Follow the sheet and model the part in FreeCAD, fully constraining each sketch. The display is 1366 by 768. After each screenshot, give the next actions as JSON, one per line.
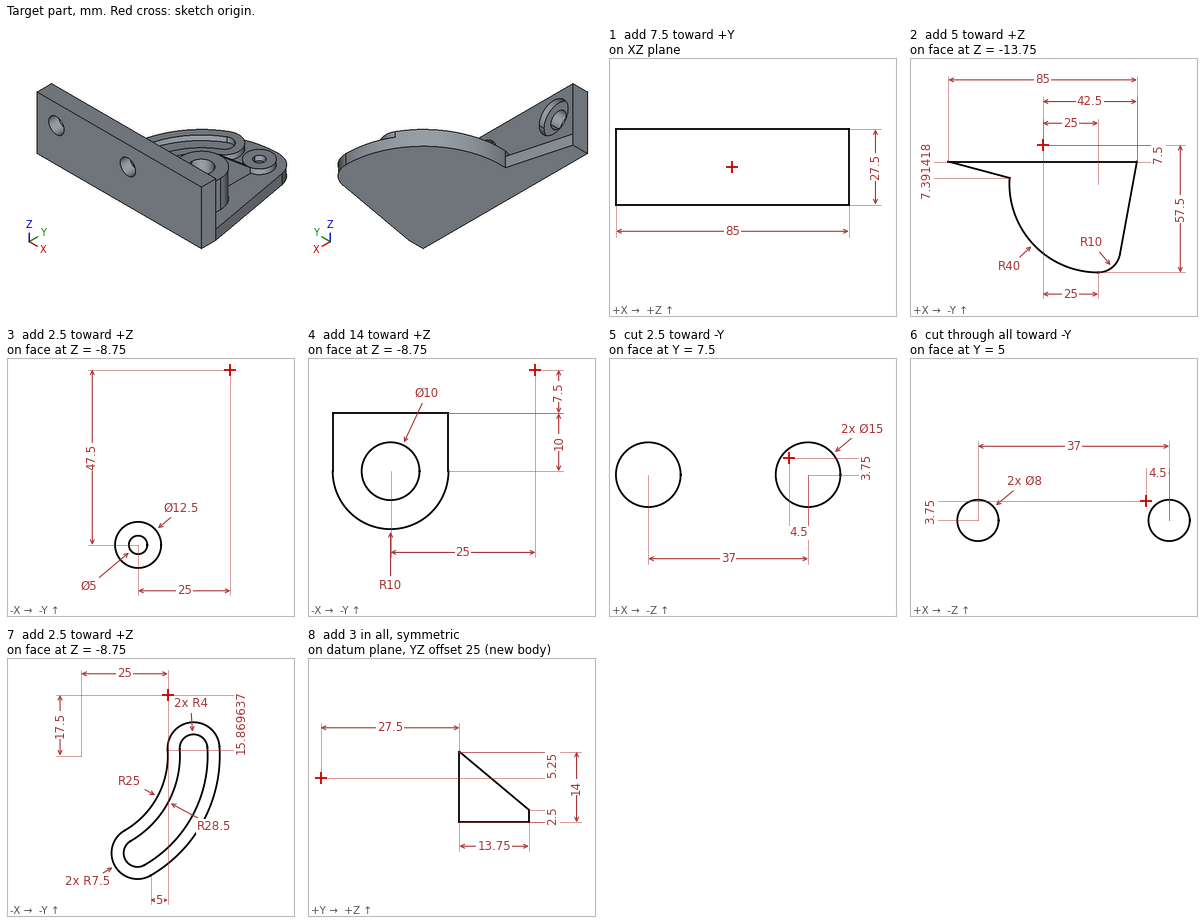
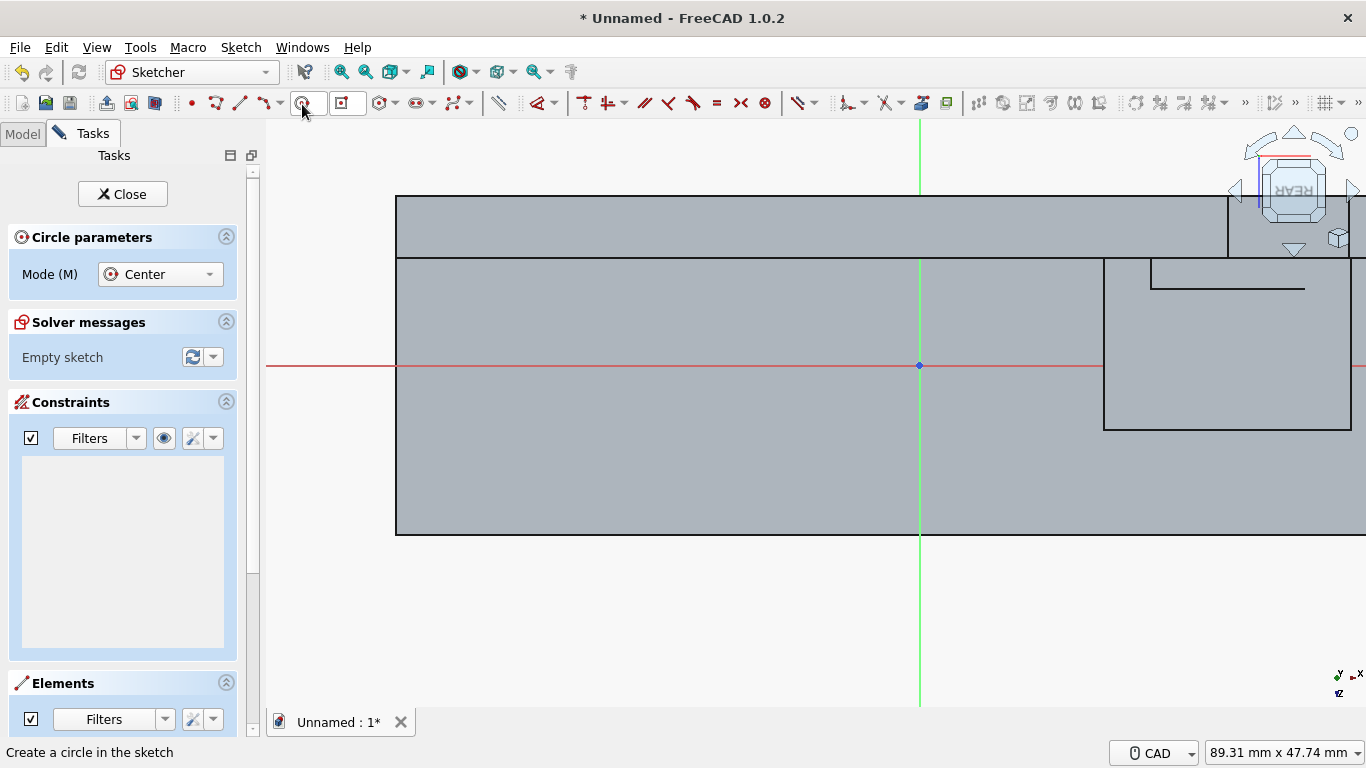
{"action": "left_click", "coordinate": [975, 412]}
{"action": "mouse_move", "coordinate": [1040, 347]}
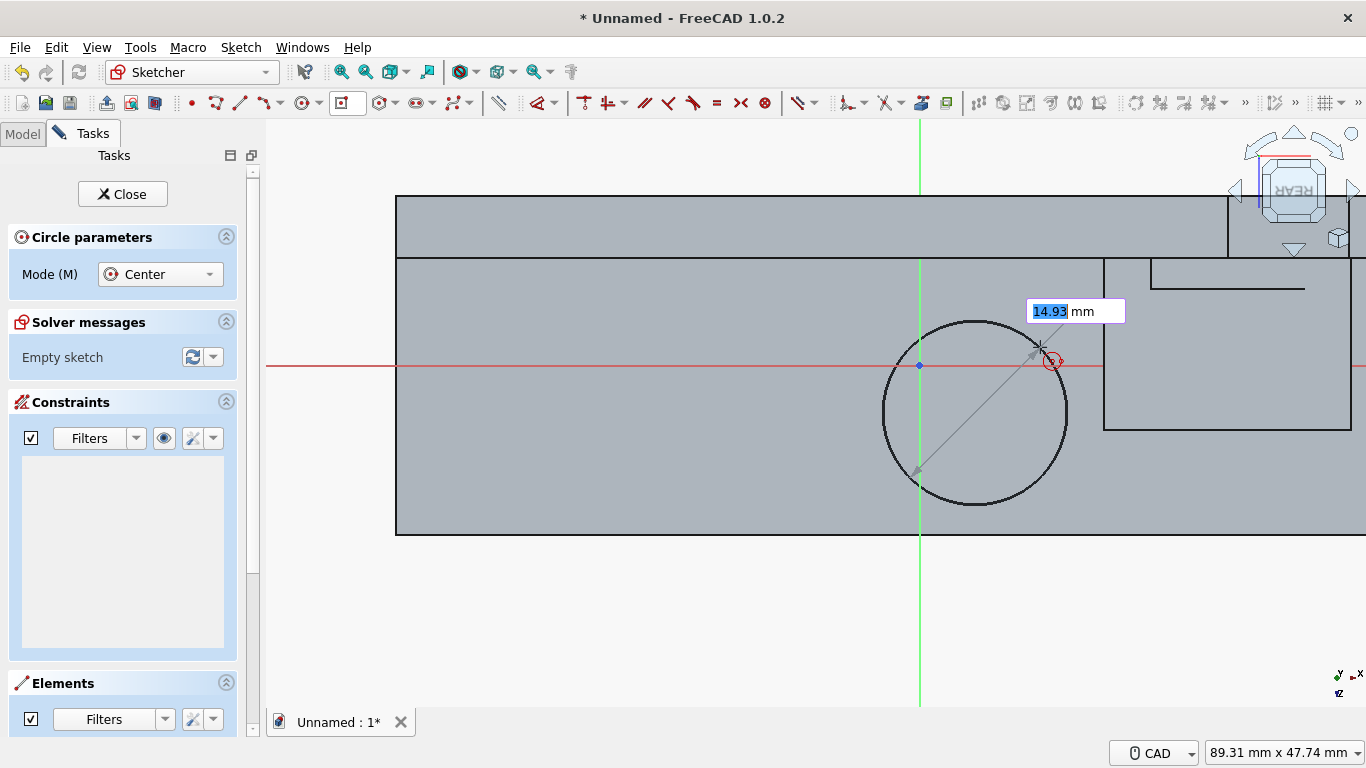
{"action": "type", "text": "15"}
{"action": "key", "text": "Return"}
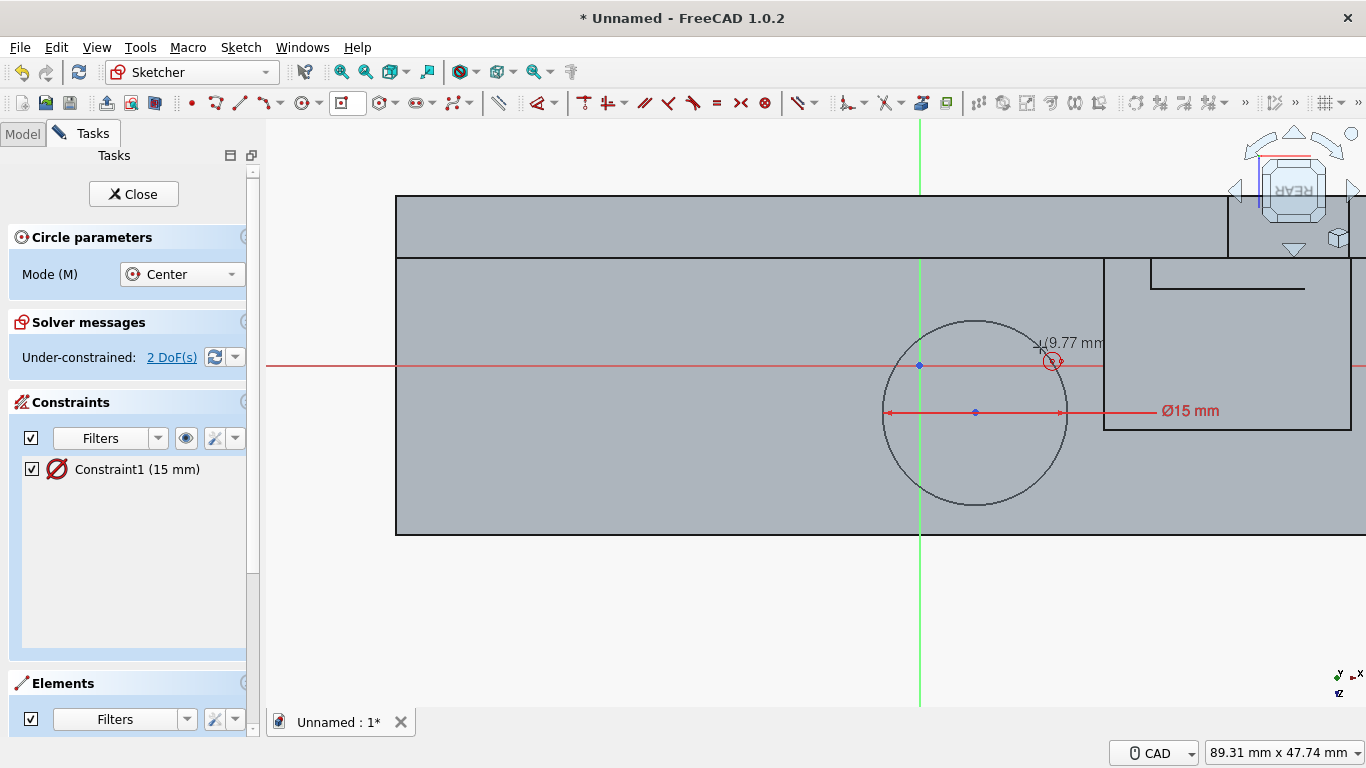
{"action": "left_click", "coordinate": [519, 412]}
{"action": "mouse_move", "coordinate": [585, 347]}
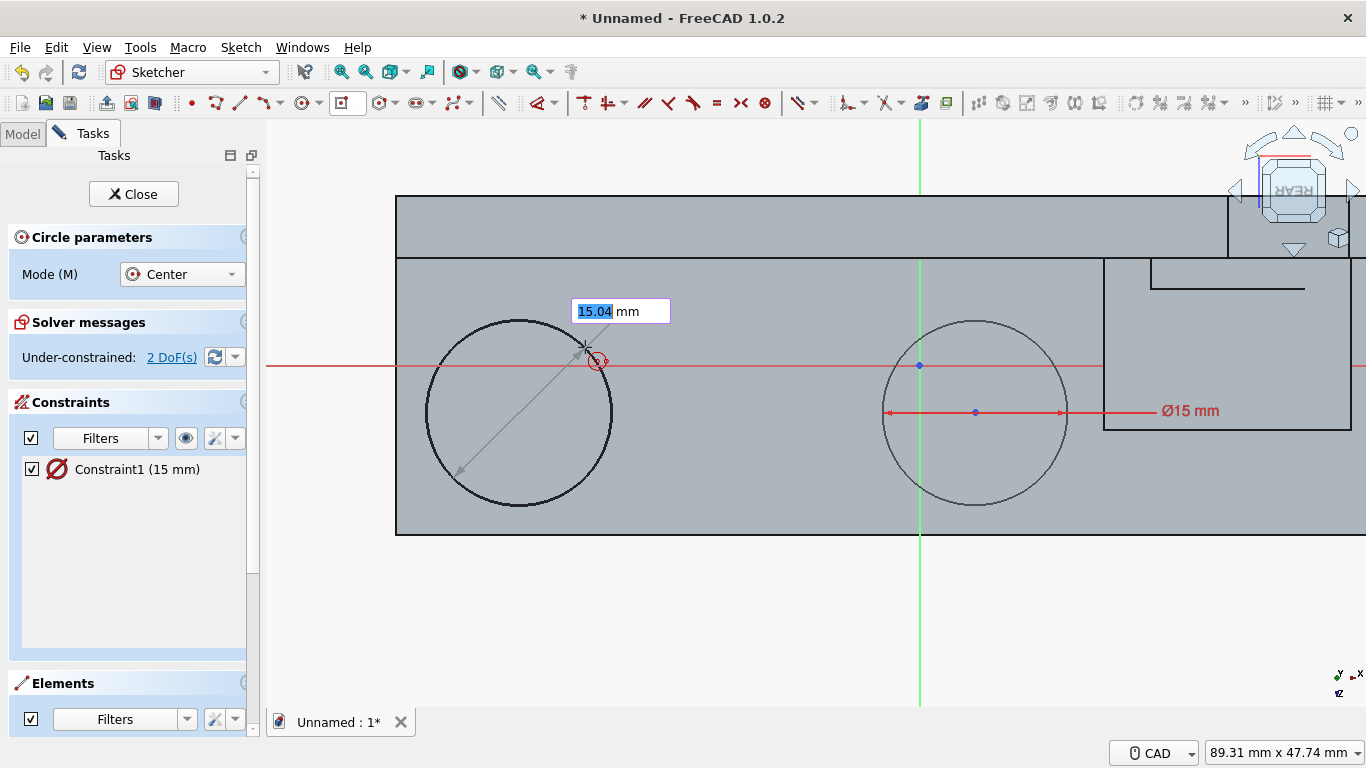
{"action": "type", "text": "15"}
{"action": "key", "text": "Return"}
{"action": "key", "text": "Escape"}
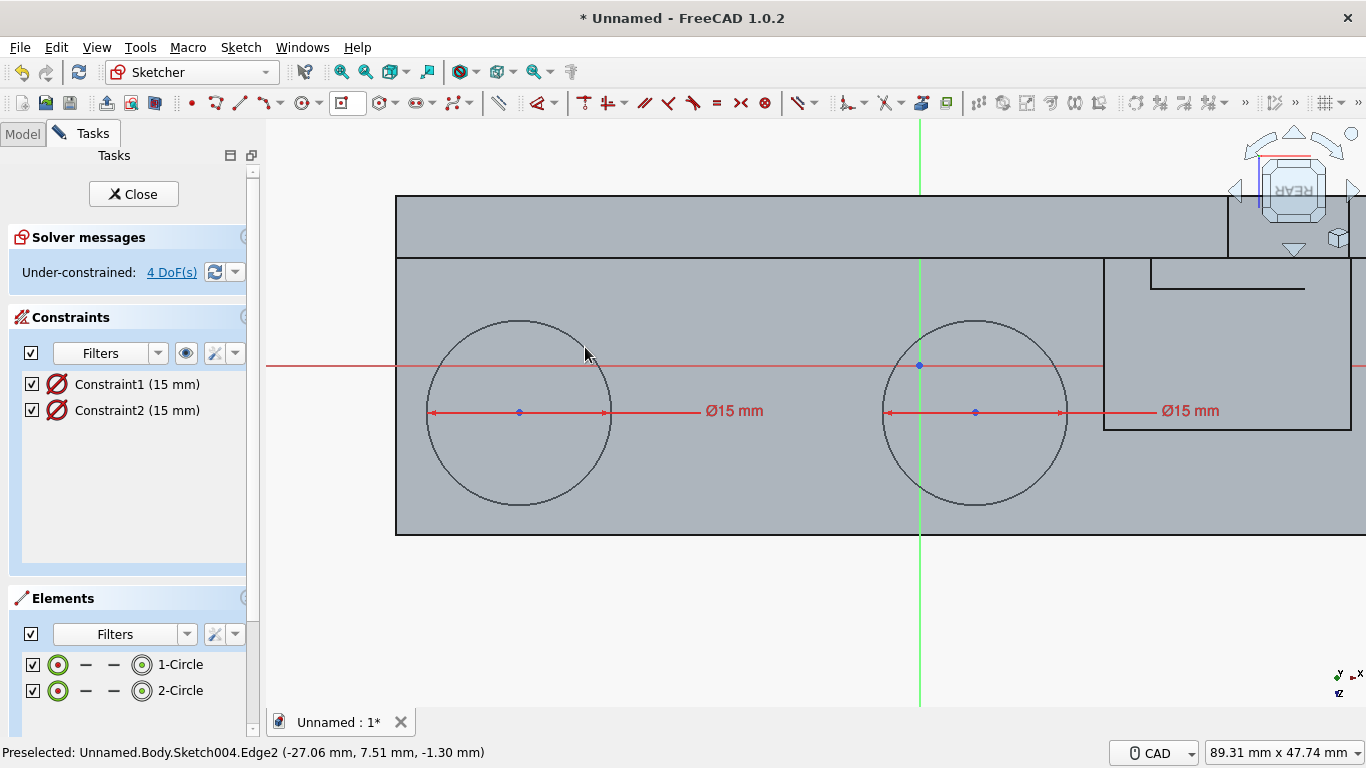
{"action": "left_click", "coordinate": [975, 413]}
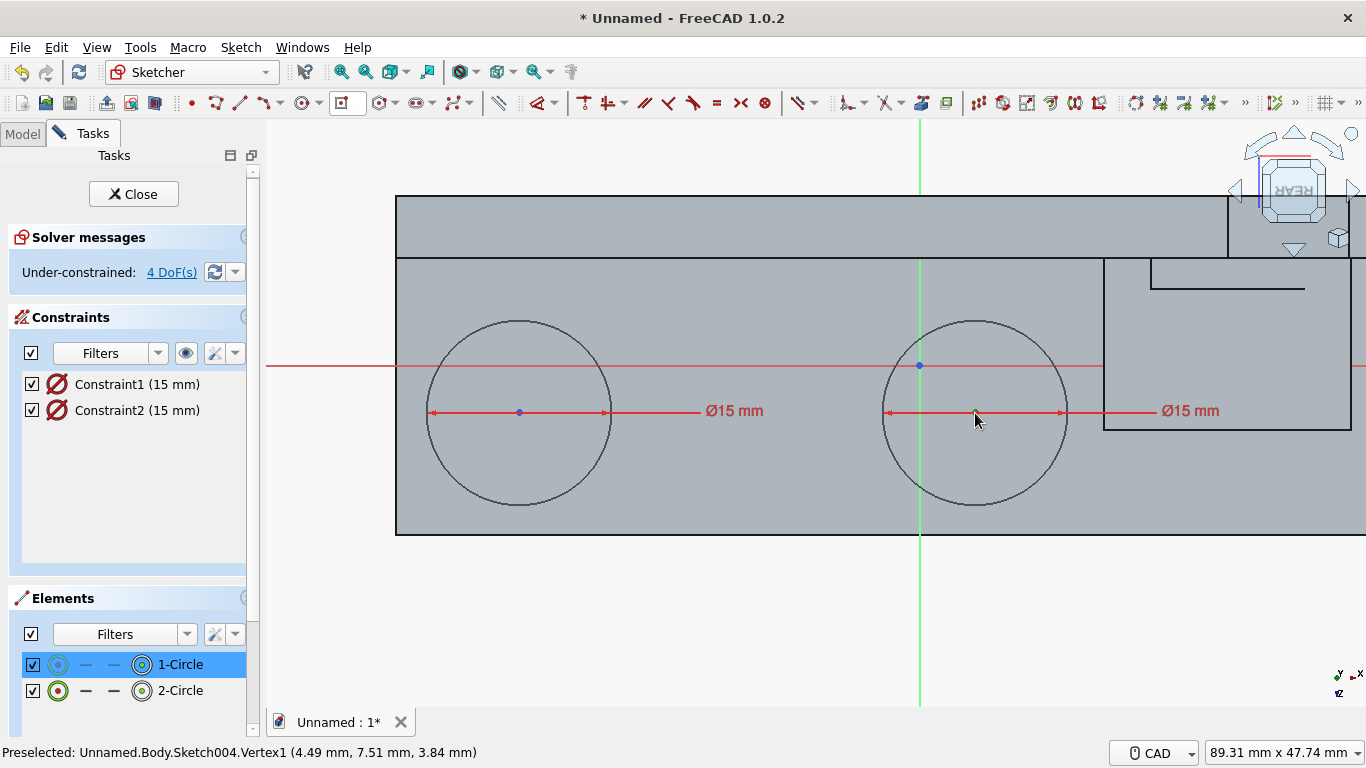
{"action": "left_click", "coordinate": [519, 413]}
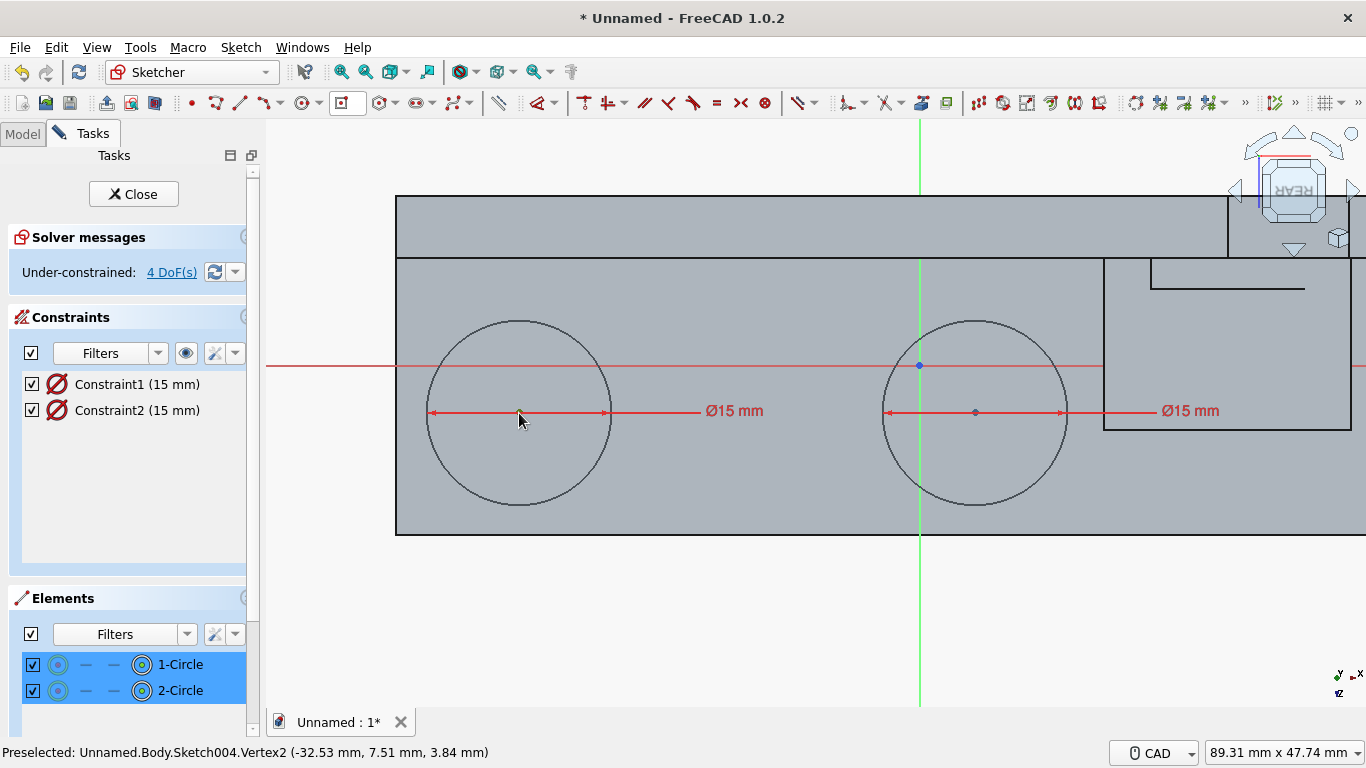
{"action": "left_click", "coordinate": [626, 104]}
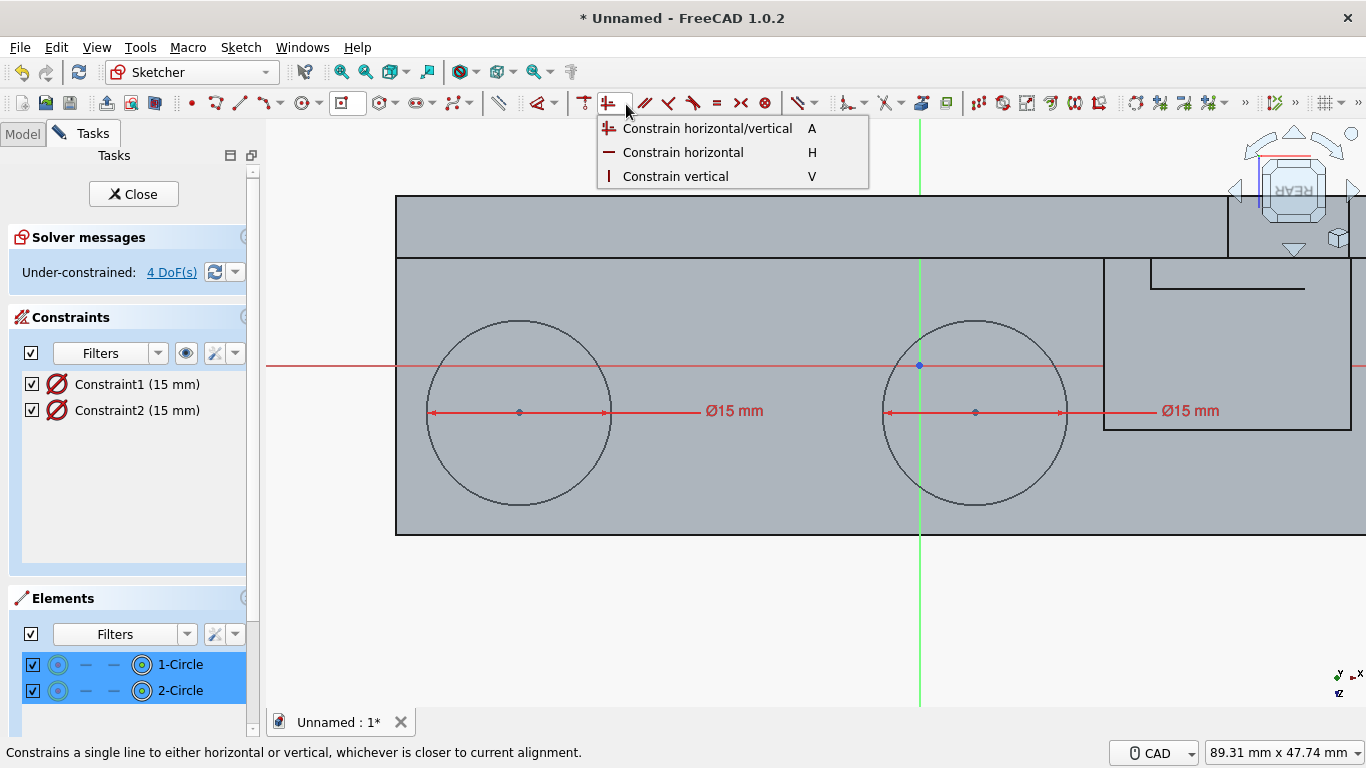
{"action": "left_click", "coordinate": [733, 152]}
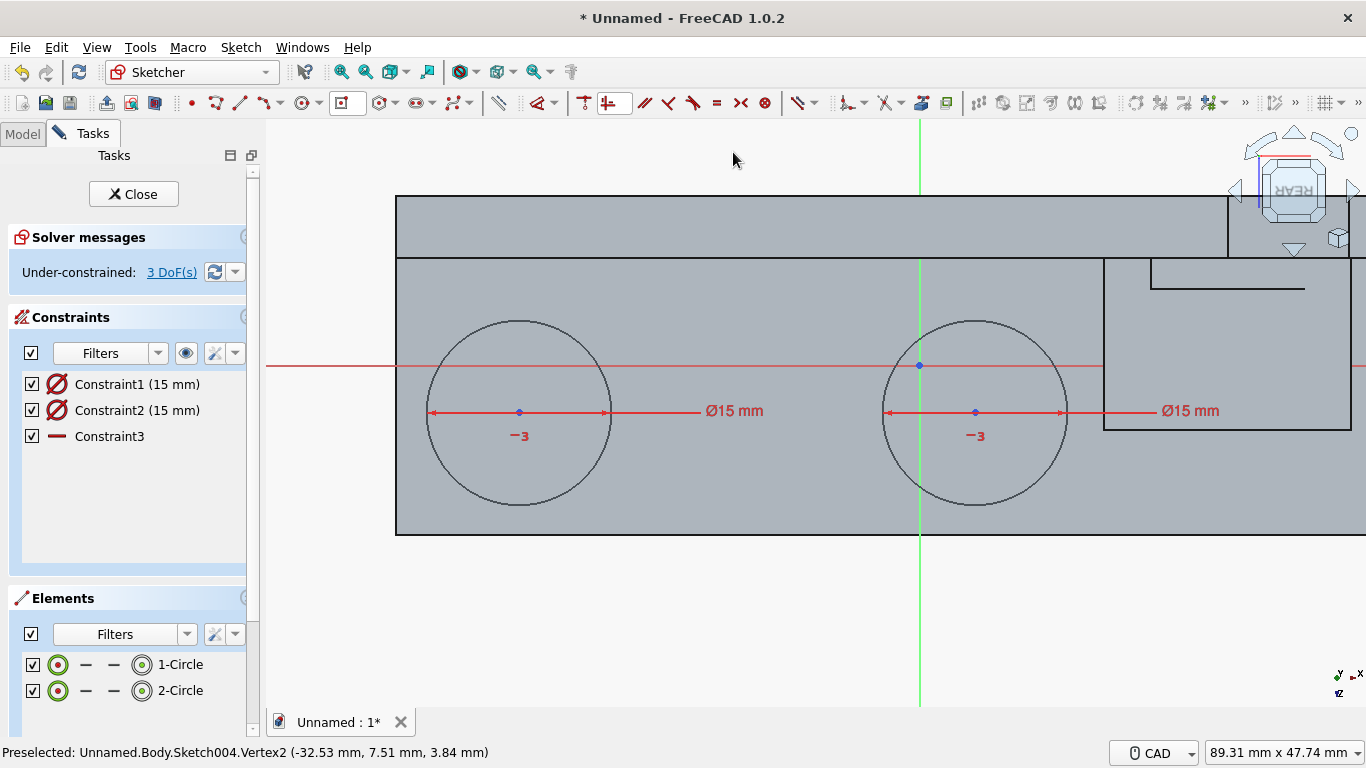
{"action": "left_click", "coordinate": [538, 104]}